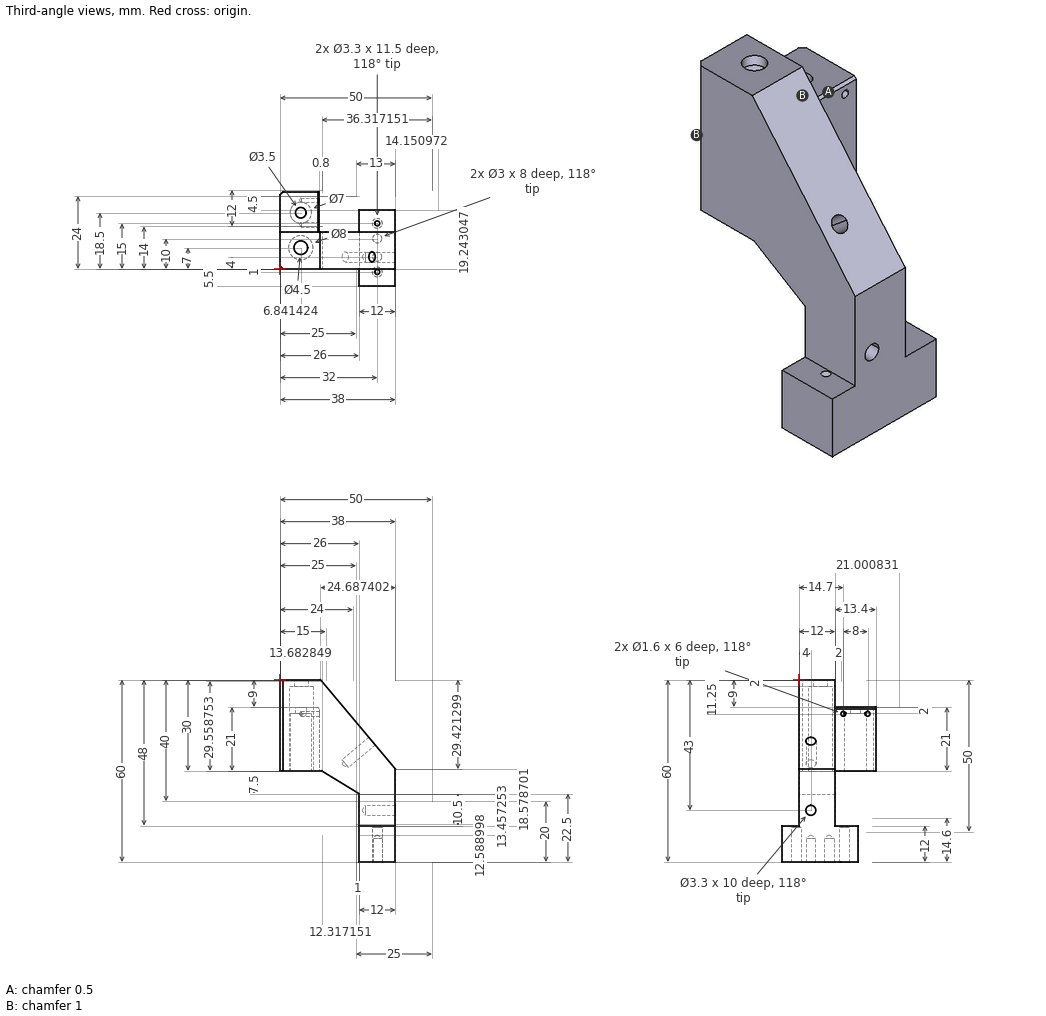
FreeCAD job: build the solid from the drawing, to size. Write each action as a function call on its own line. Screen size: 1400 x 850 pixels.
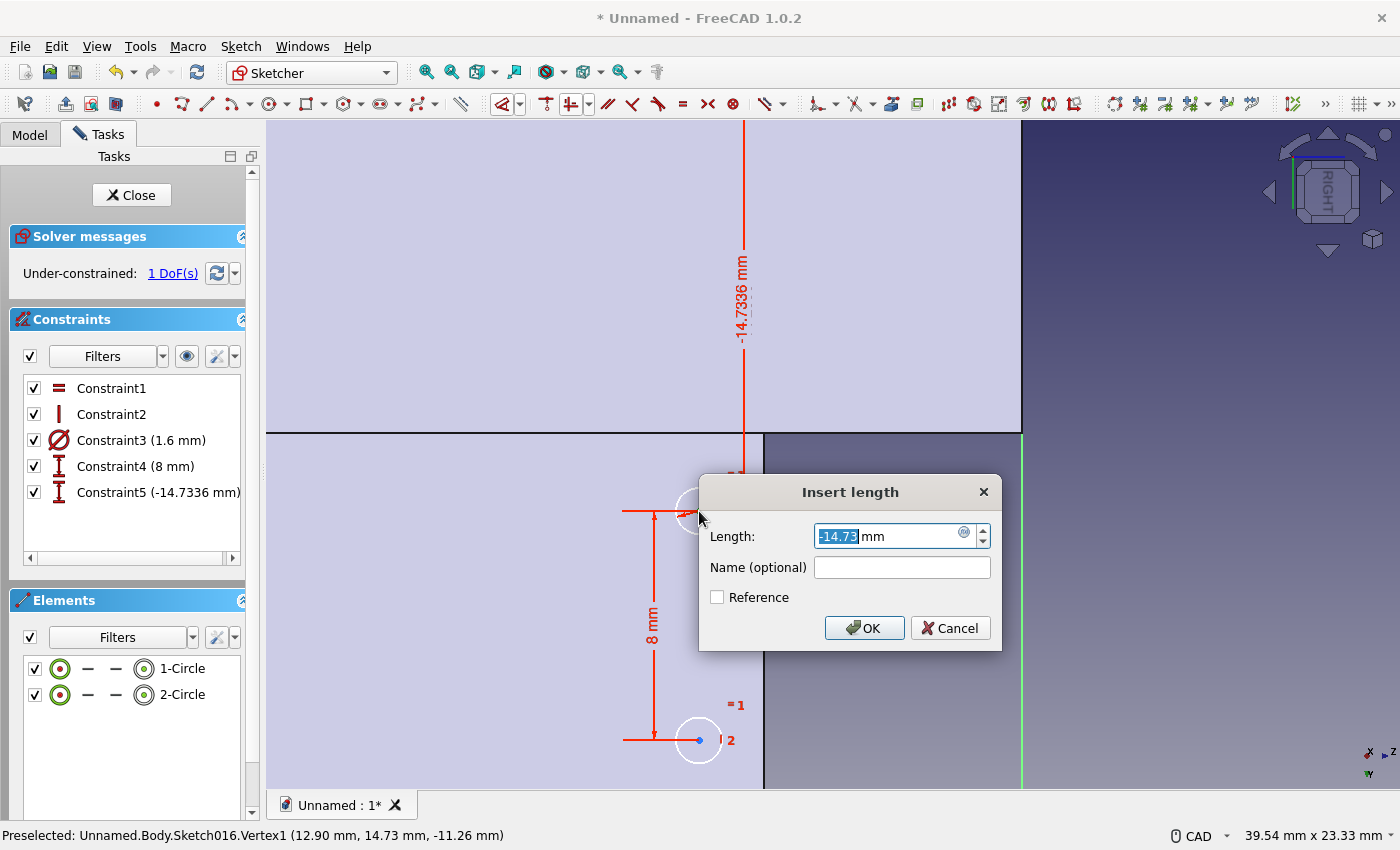
text(-14.7)
key(Return)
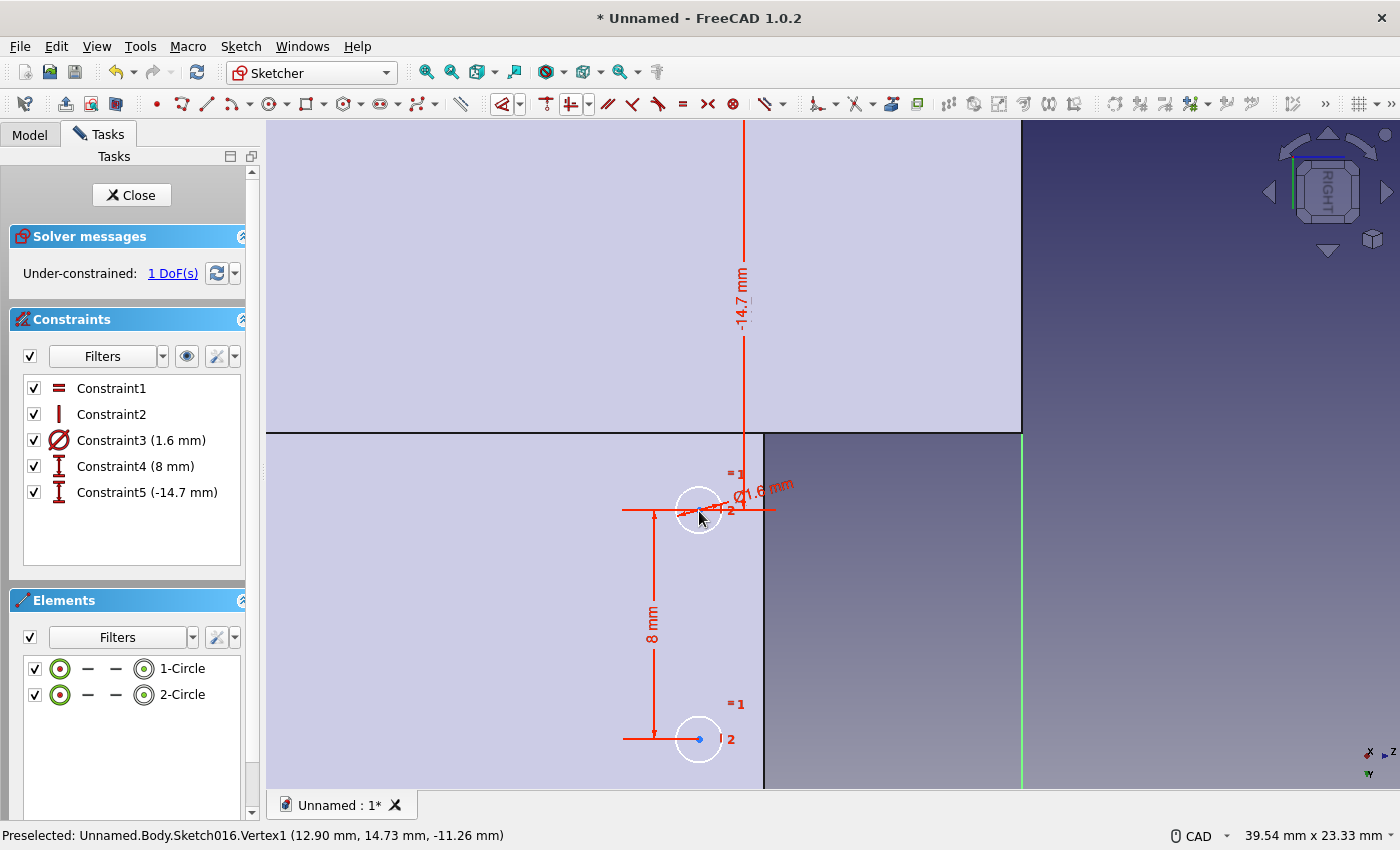
click(699, 510)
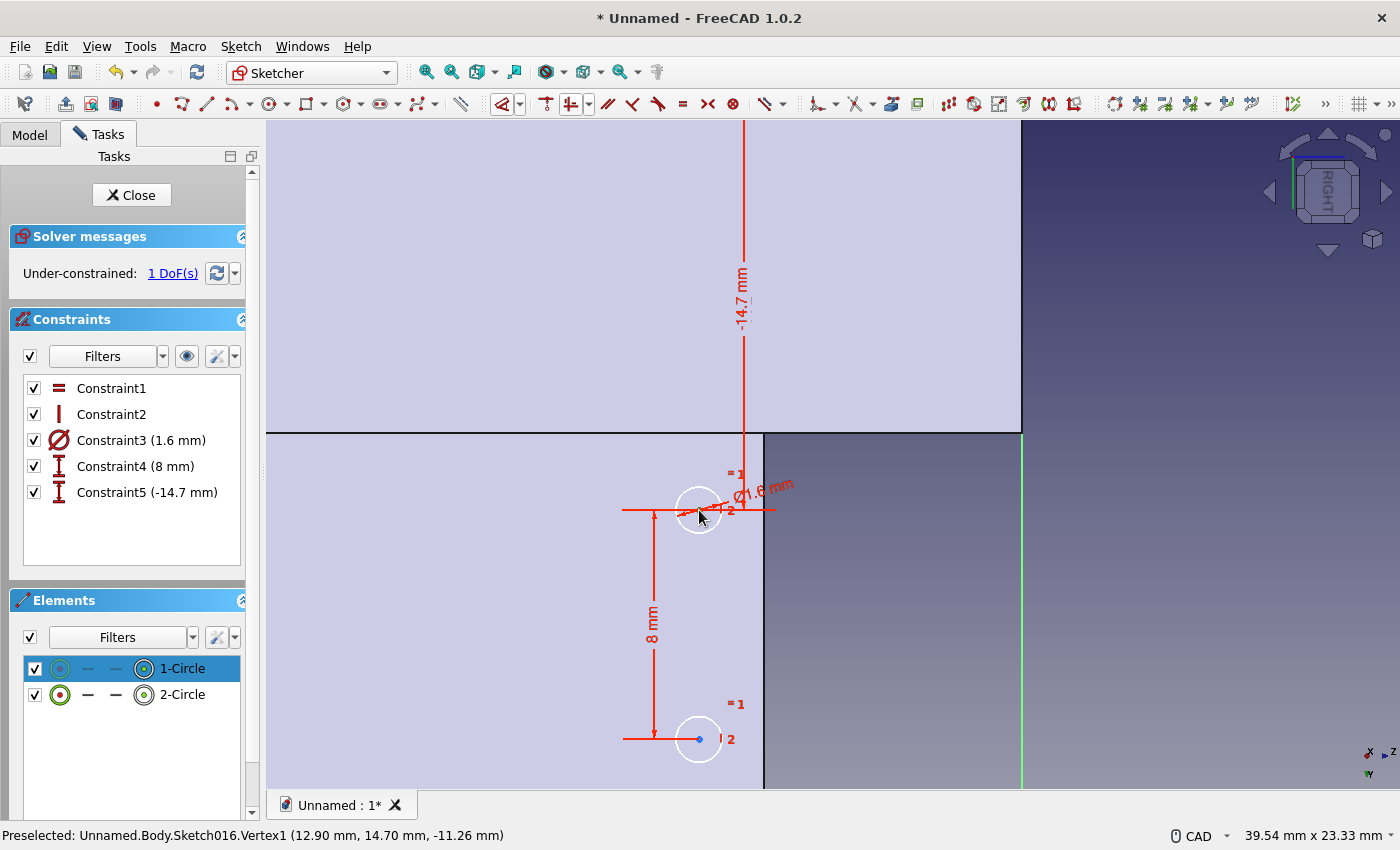
click(520, 104)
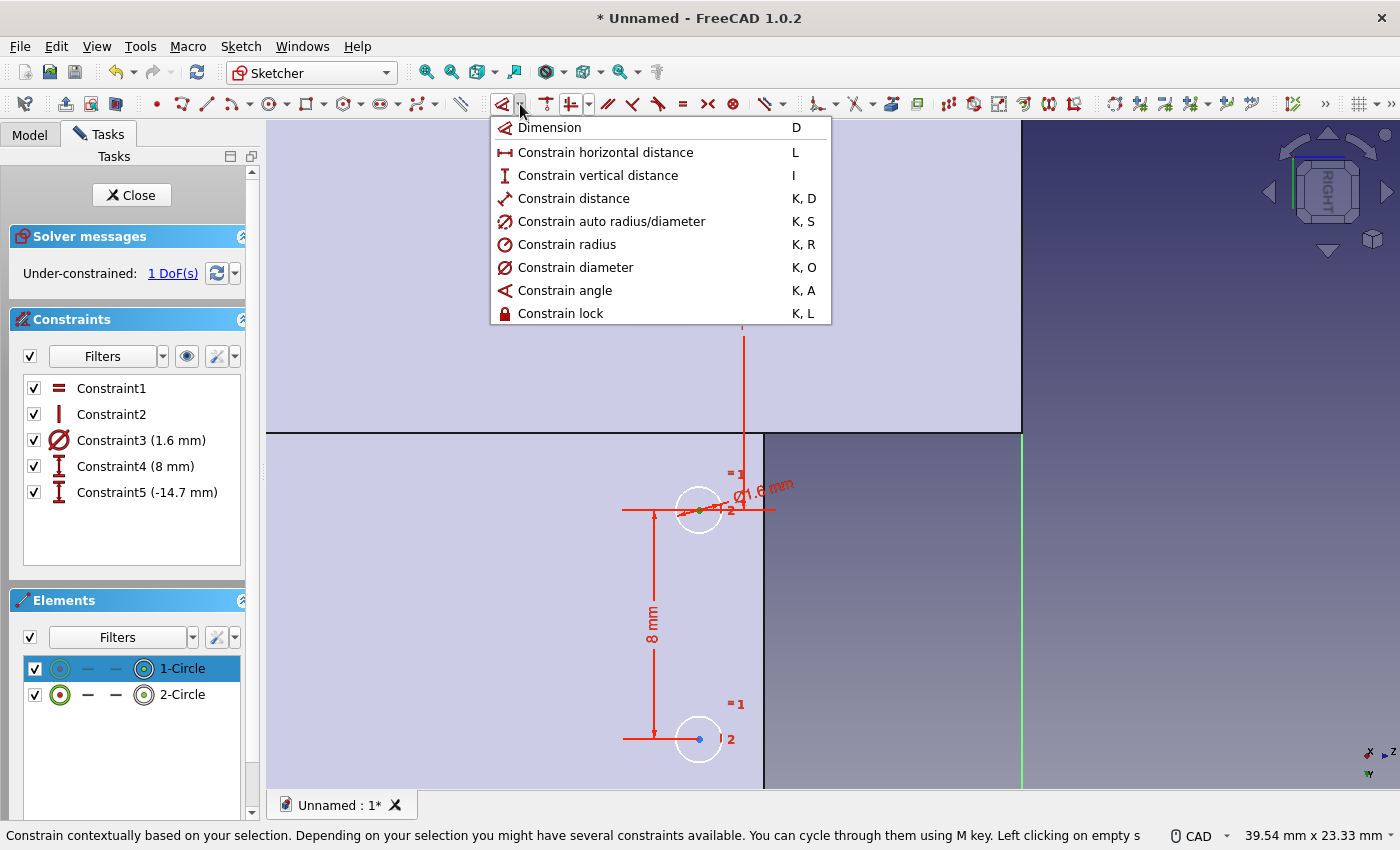
click(661, 152)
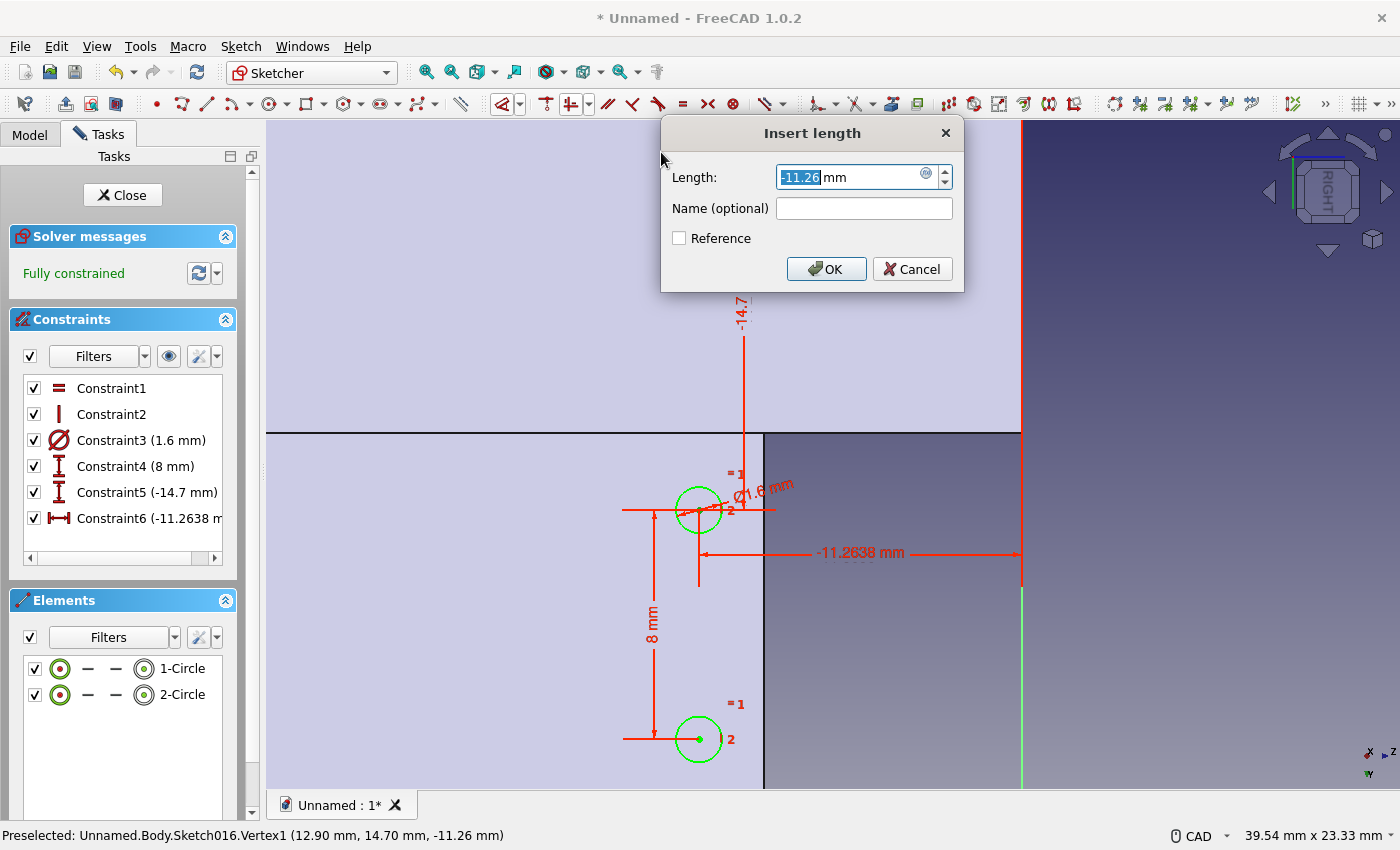
text(-11.25)
key(Return)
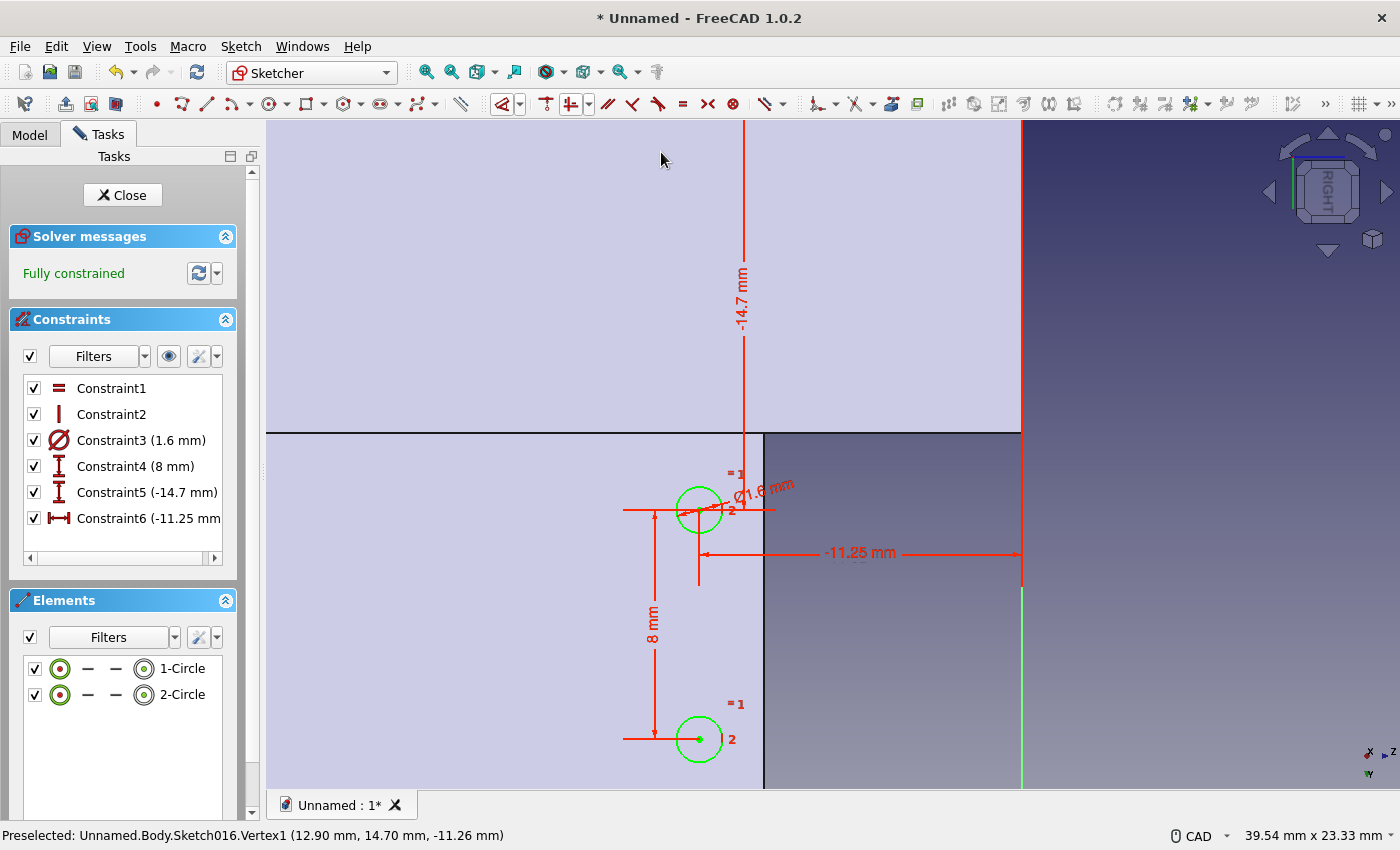
click(123, 195)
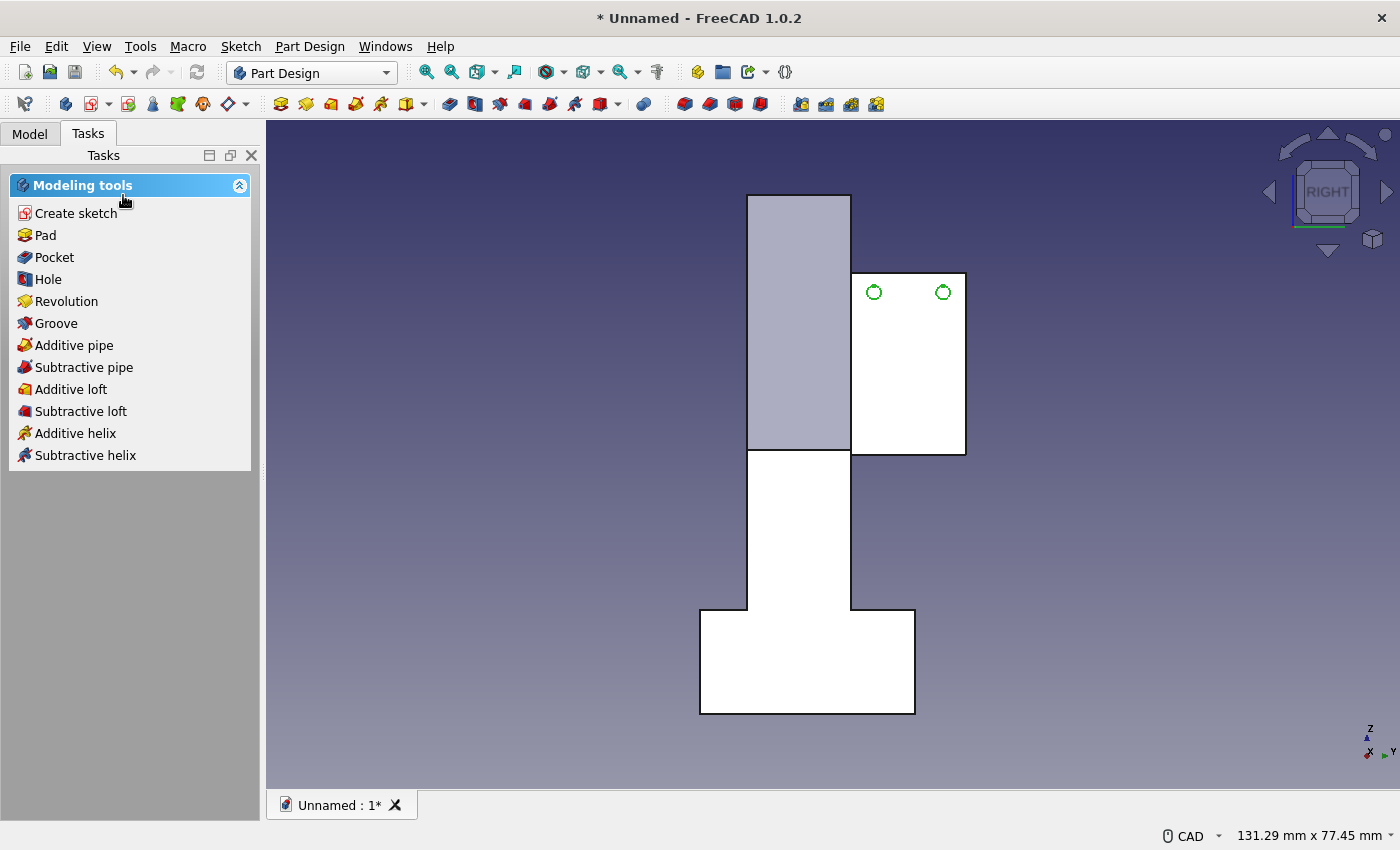
click(475, 104)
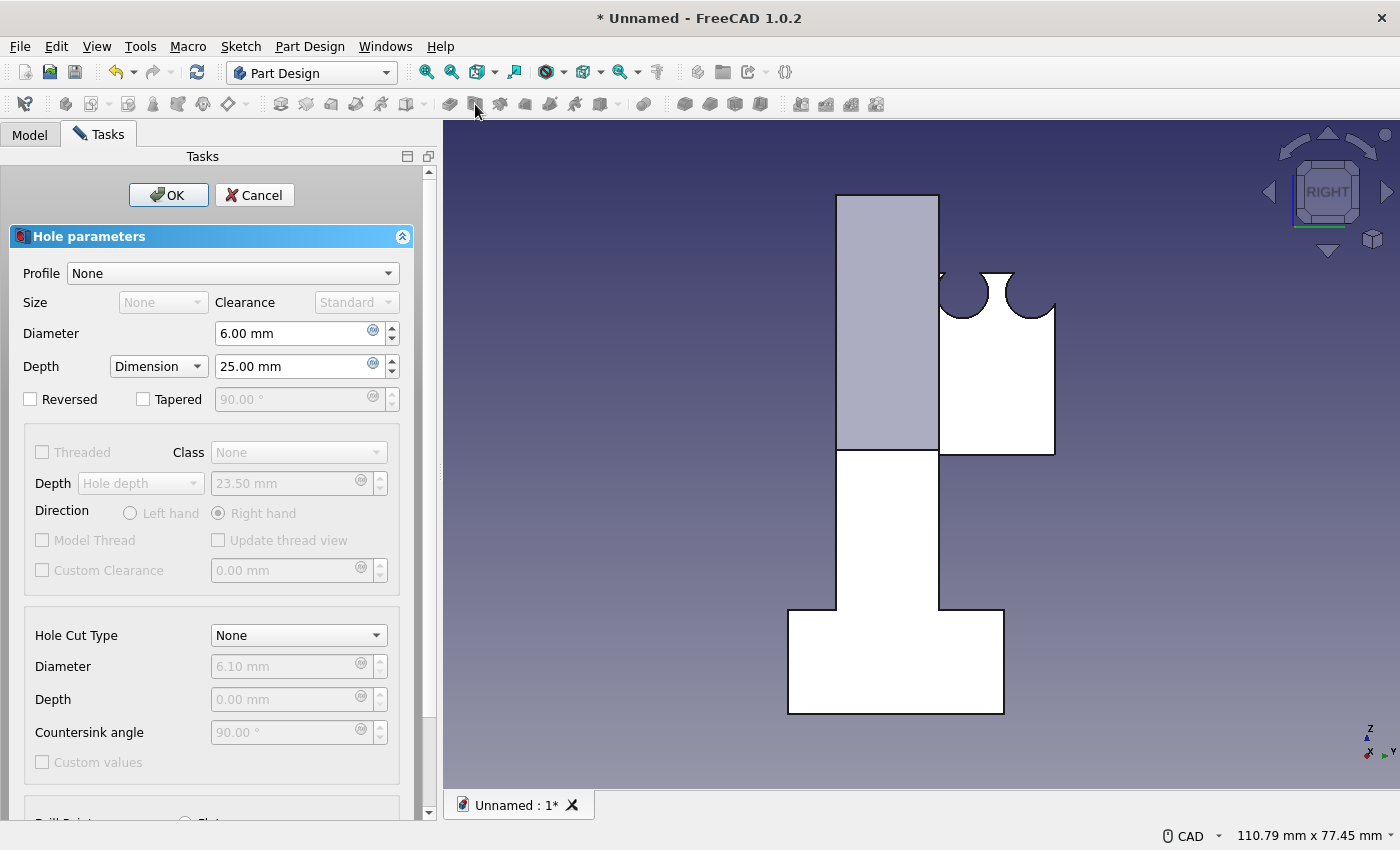
triple_click(300, 334)